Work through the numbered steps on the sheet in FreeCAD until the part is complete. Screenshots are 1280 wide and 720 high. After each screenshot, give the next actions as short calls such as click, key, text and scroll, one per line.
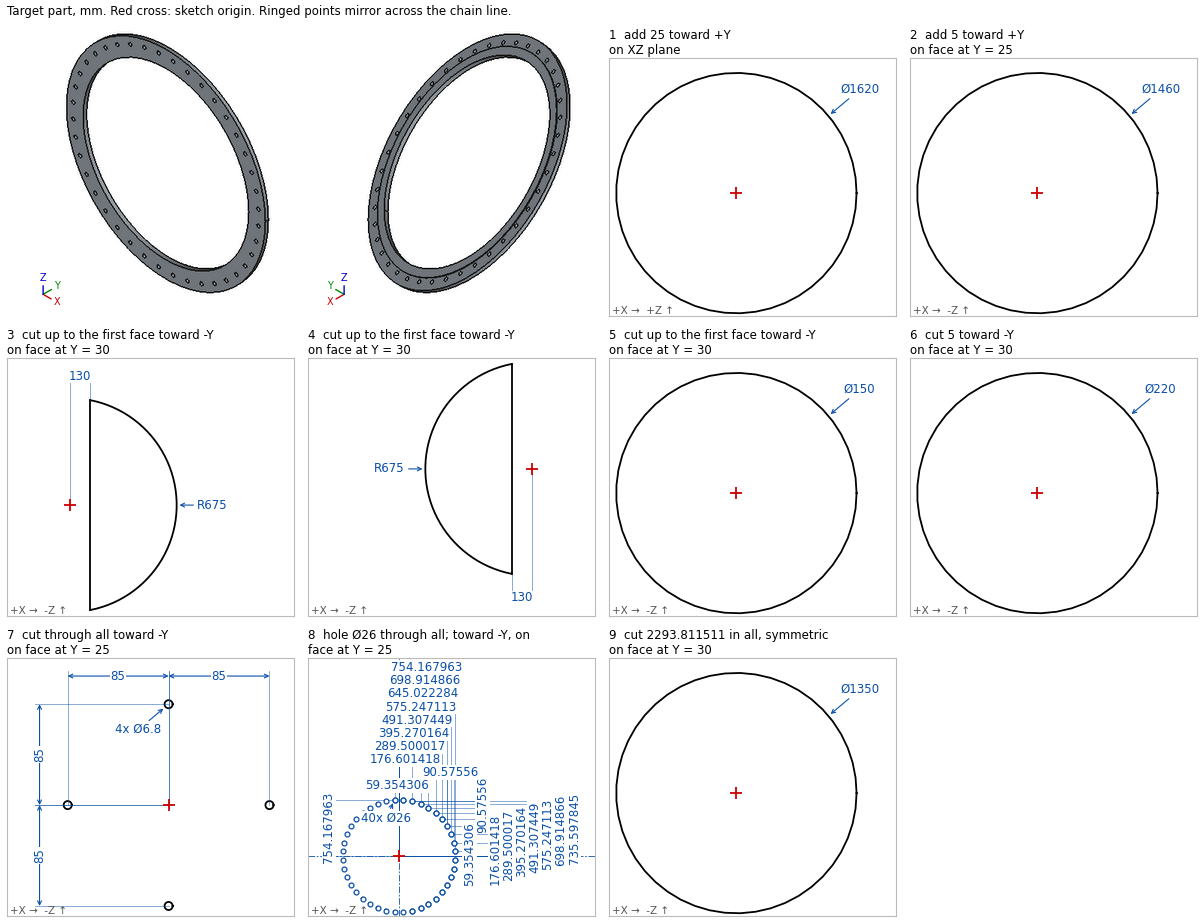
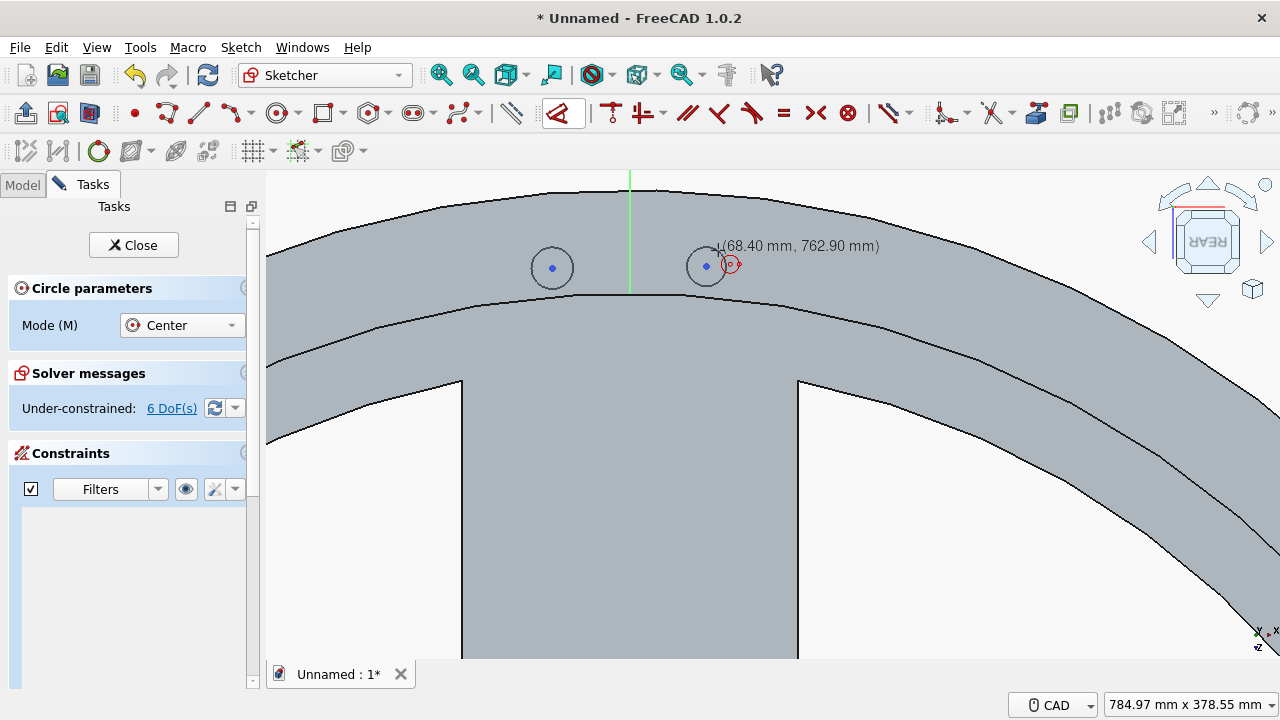
scroll(858, 286, up, 2)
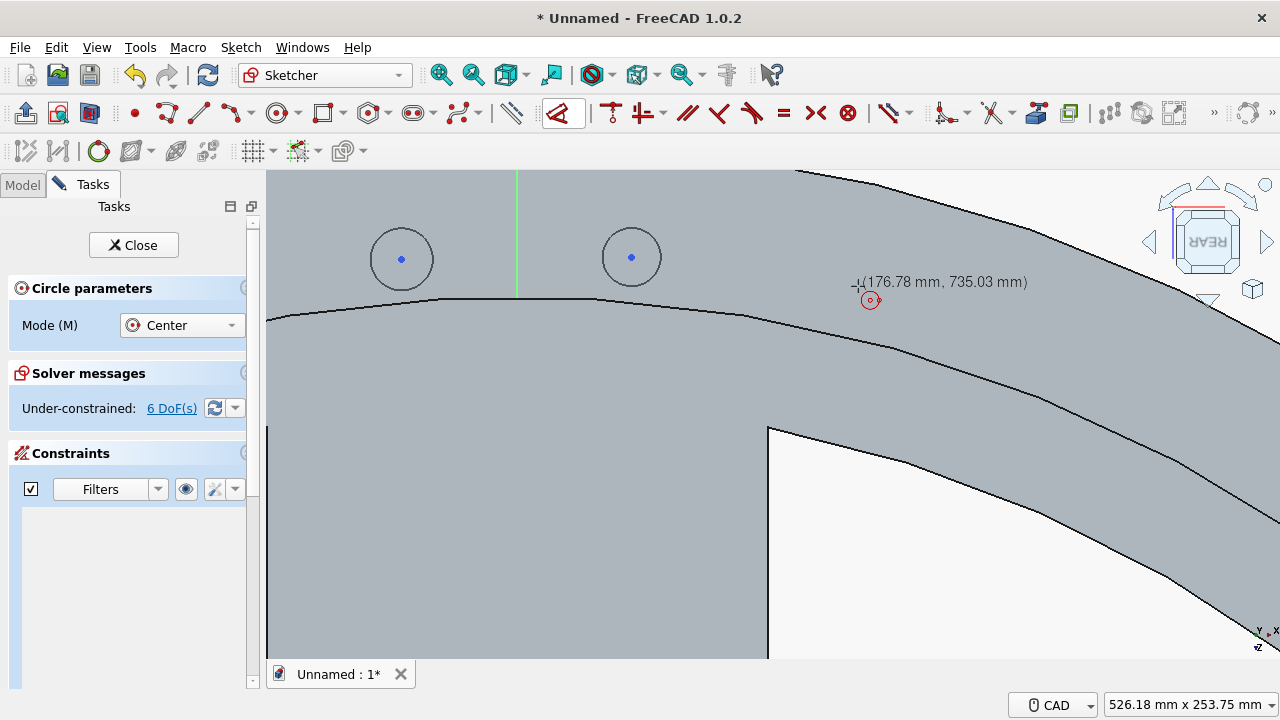
scroll(728, 254, down, 11)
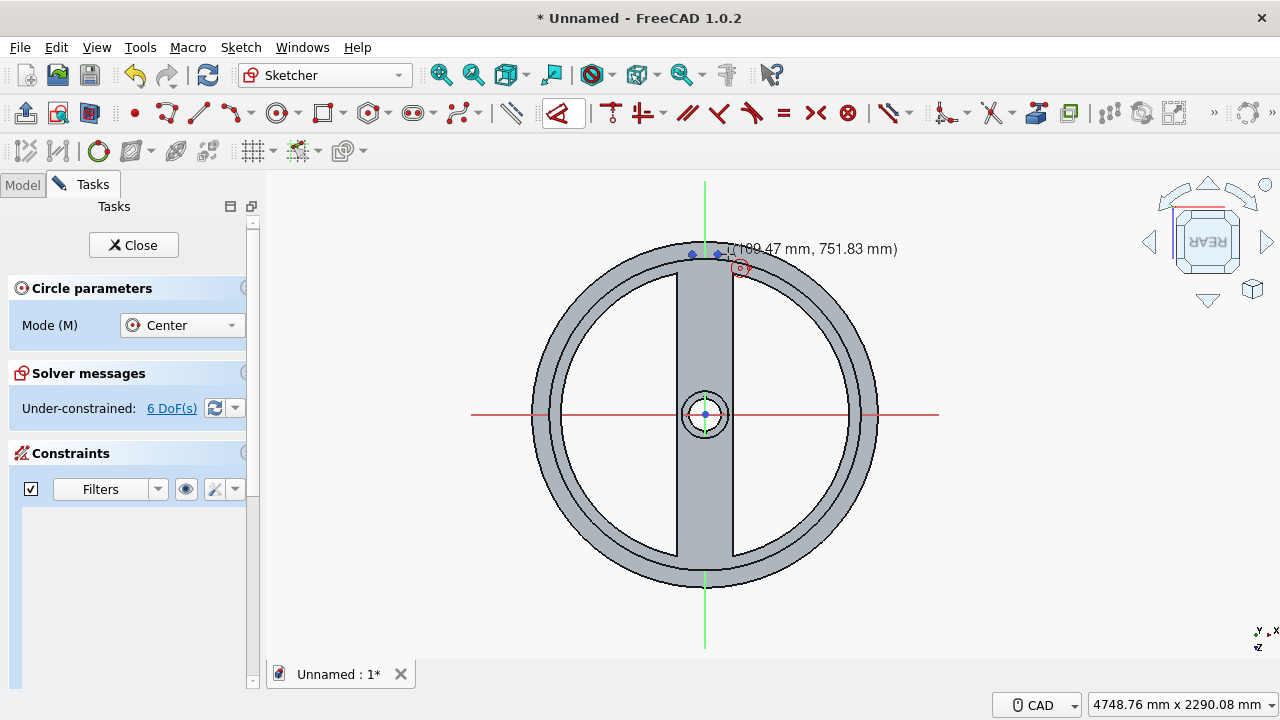
click(743, 258)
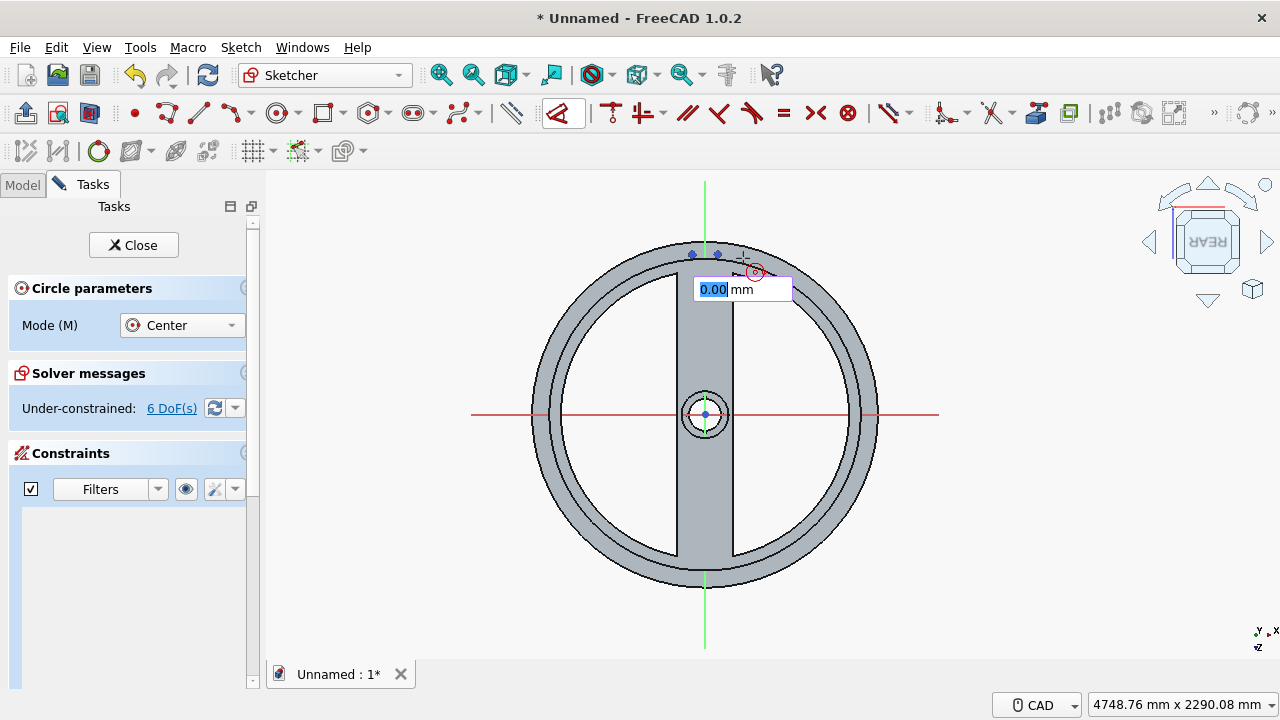
scroll(745, 256, up, 9)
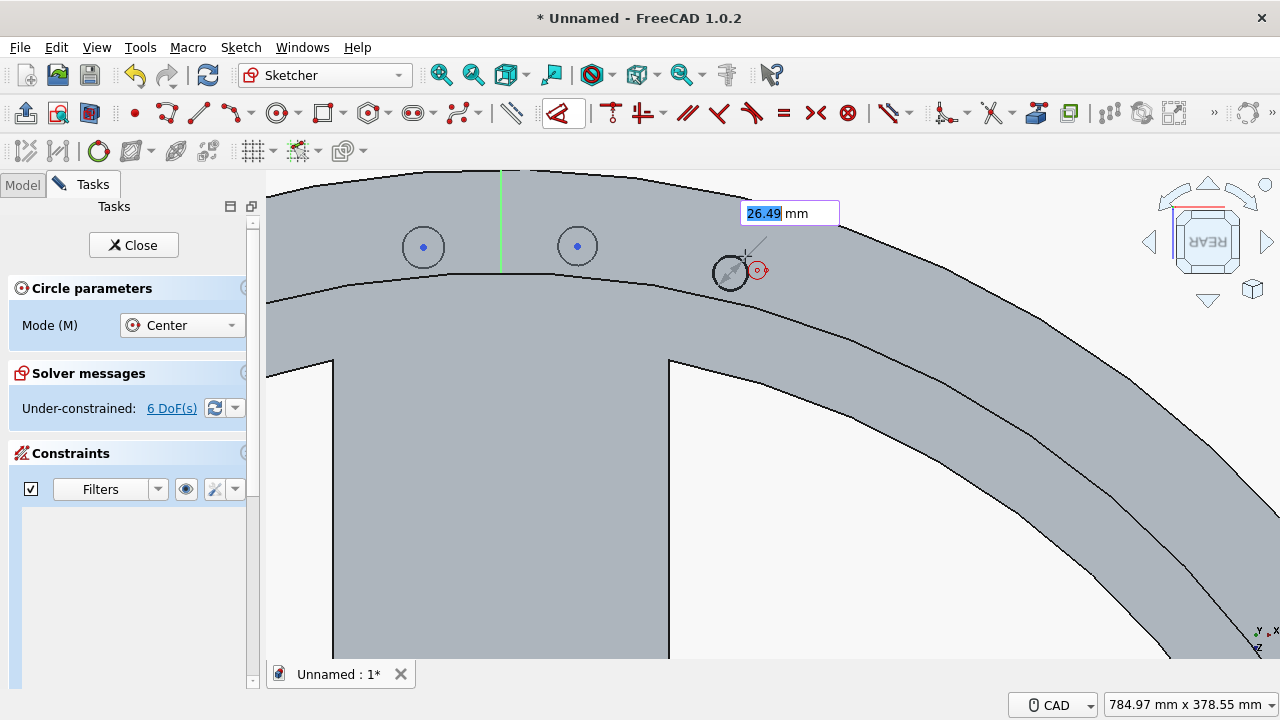
click(741, 254)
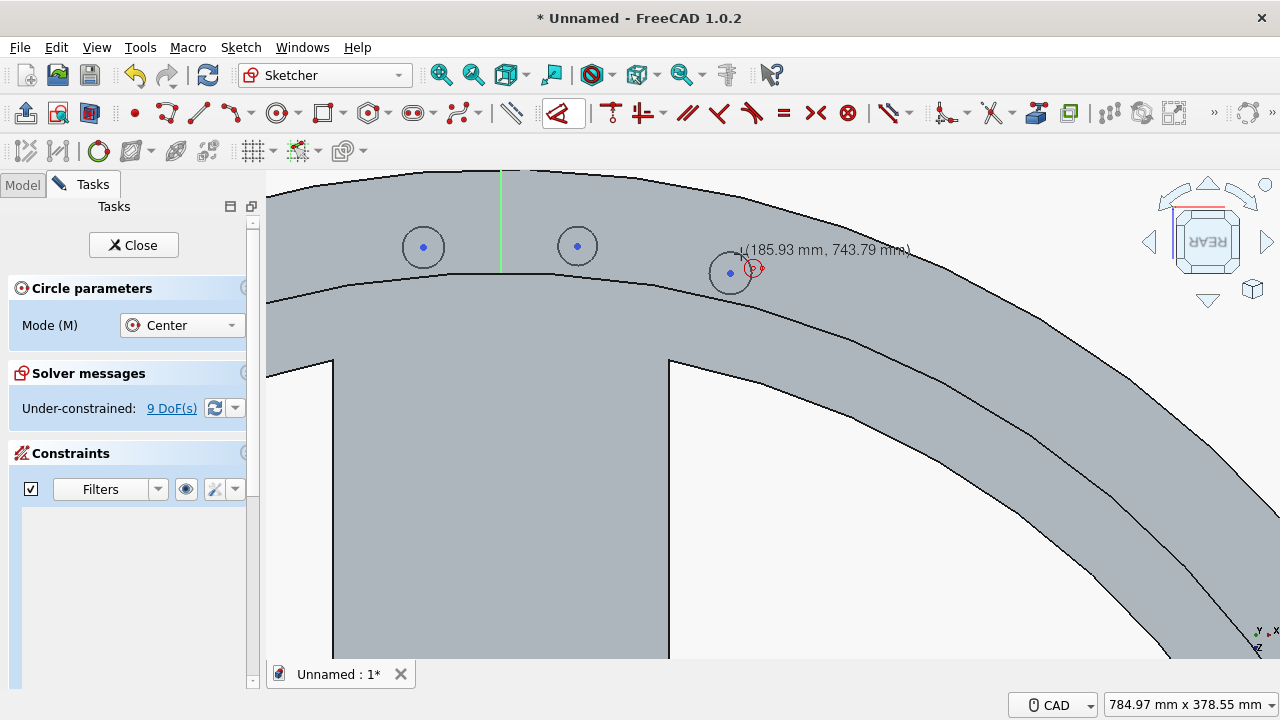
scroll(875, 313, up, 2)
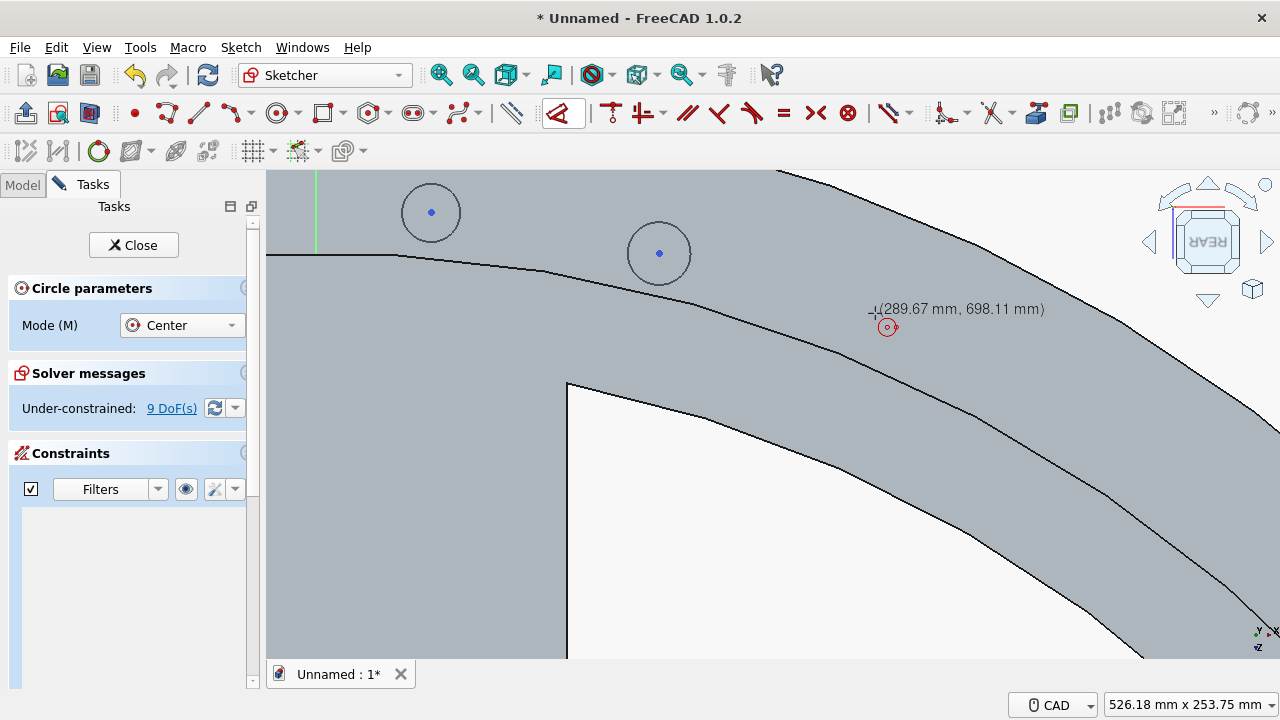
scroll(753, 259, down, 11)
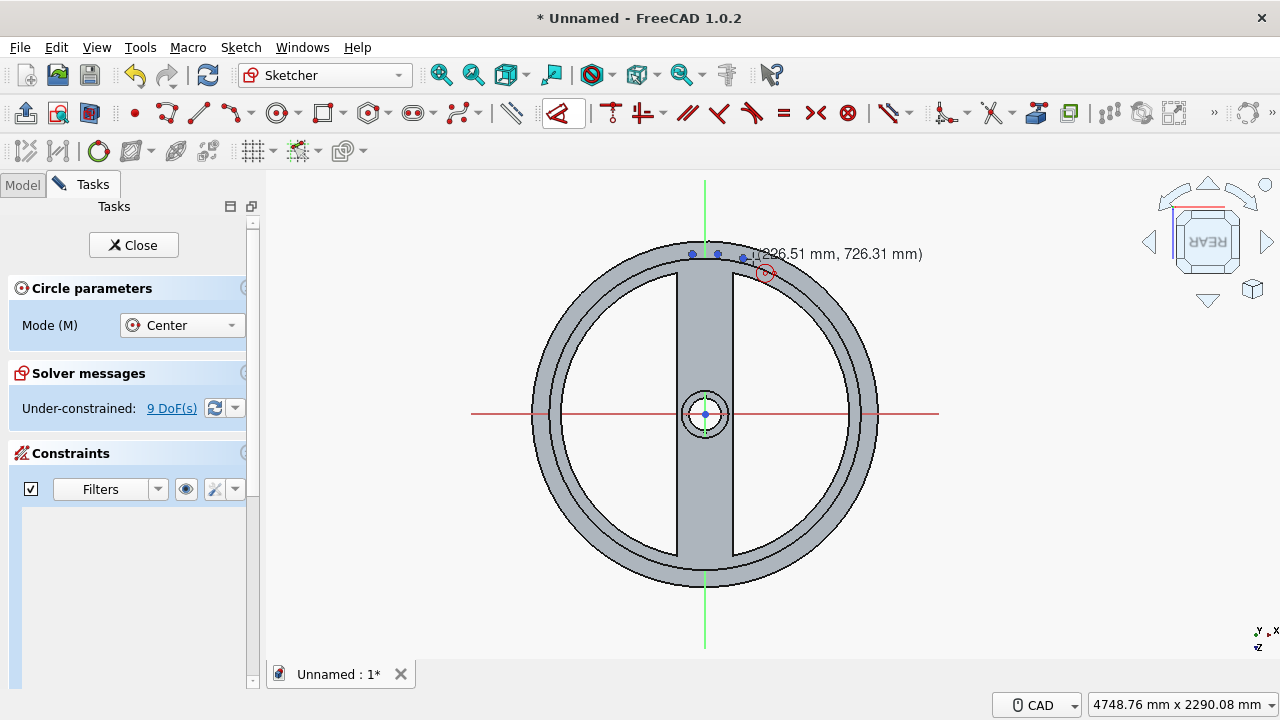
click(767, 265)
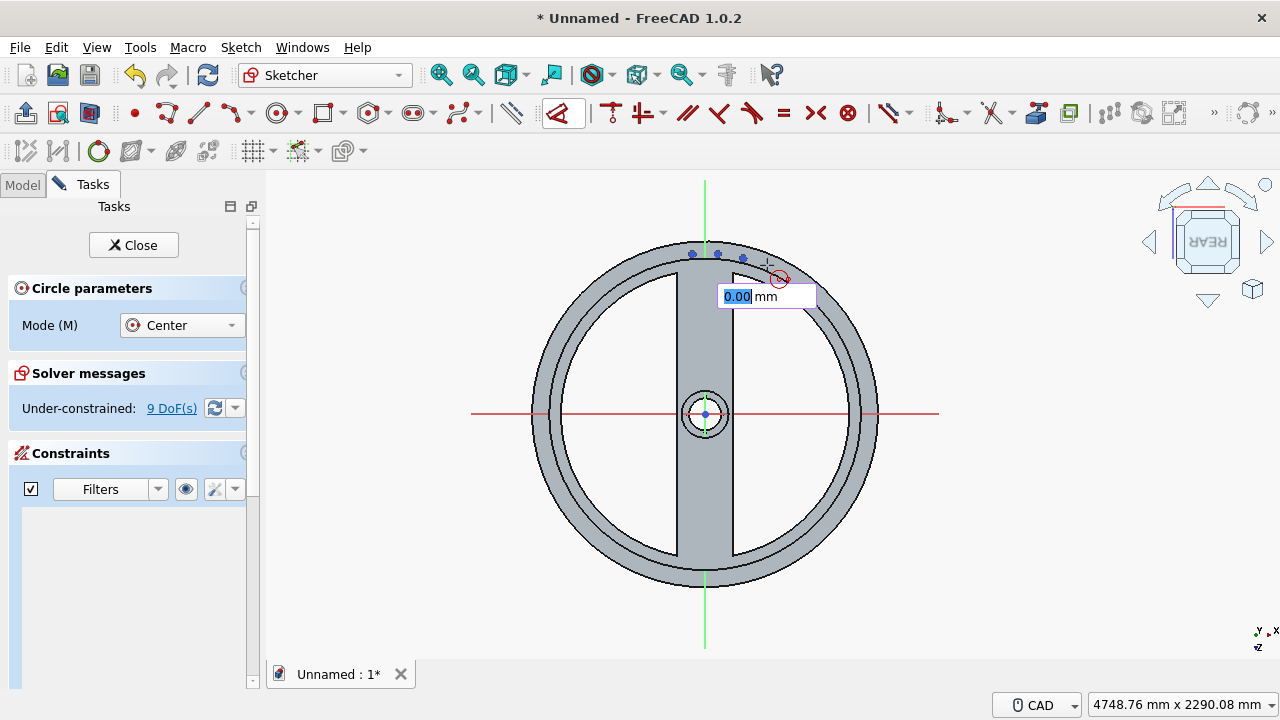
scroll(769, 263, up, 9)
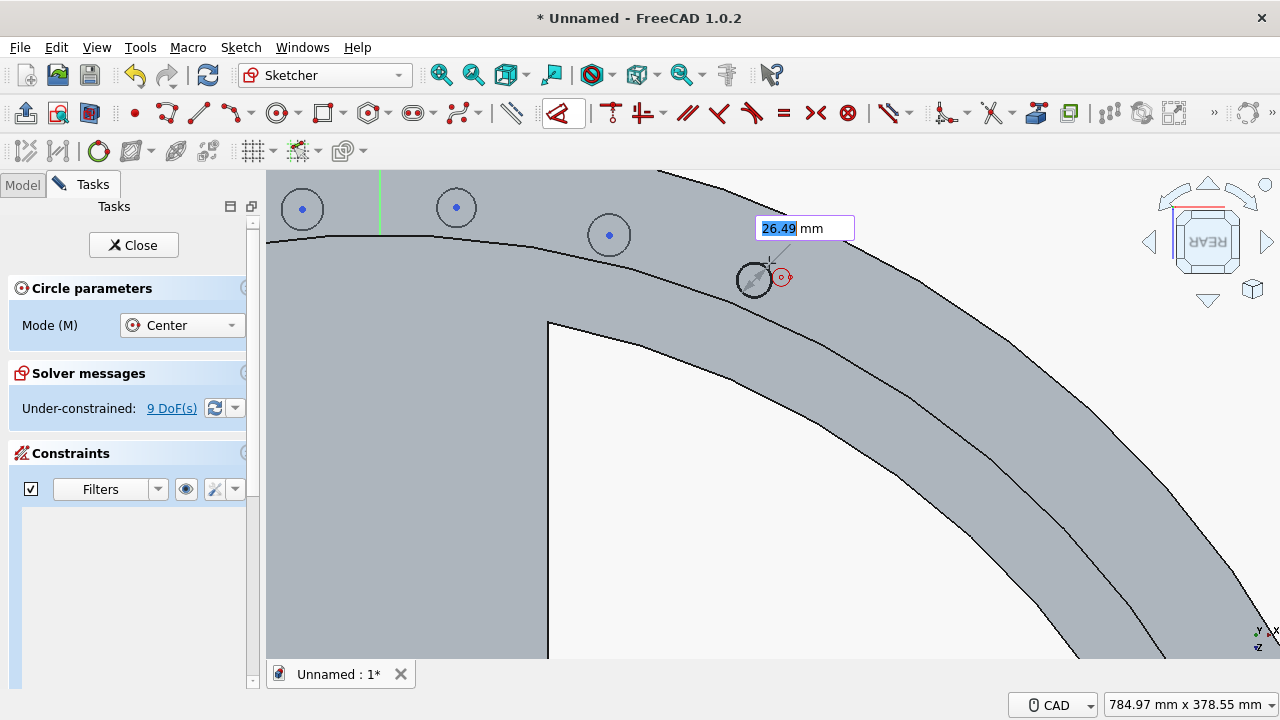
click(766, 263)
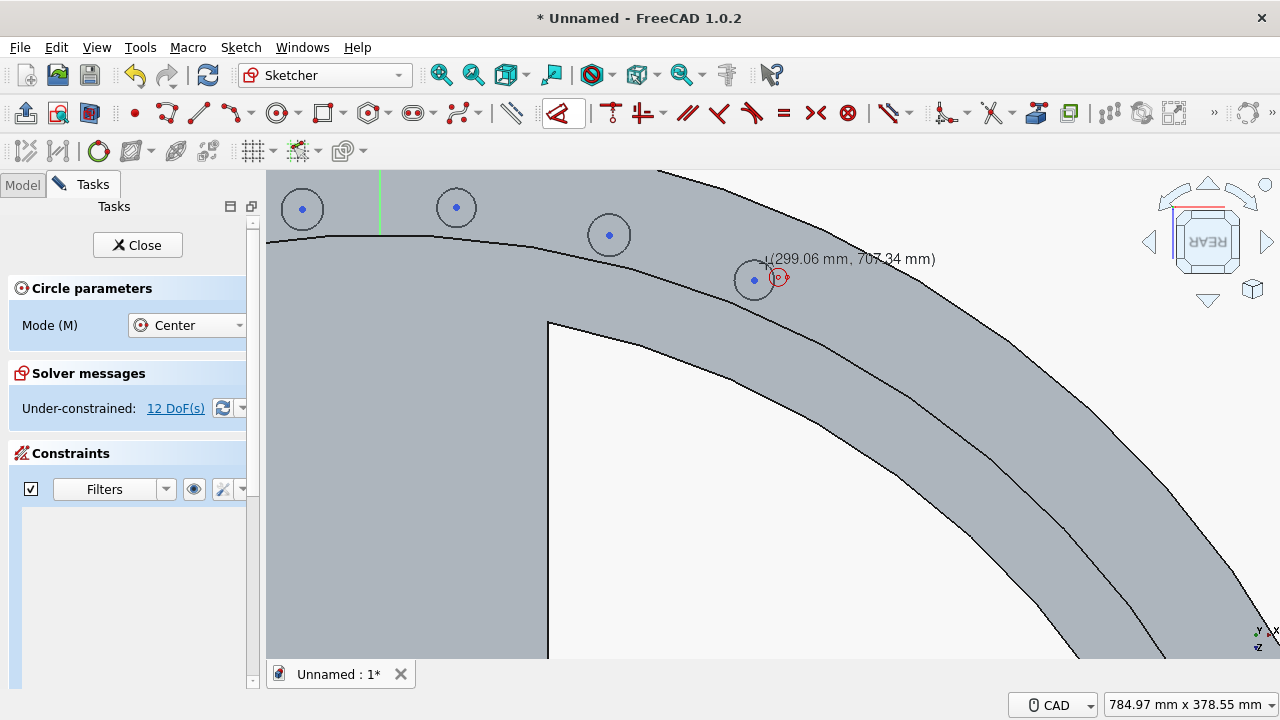
scroll(890, 345, up, 2)